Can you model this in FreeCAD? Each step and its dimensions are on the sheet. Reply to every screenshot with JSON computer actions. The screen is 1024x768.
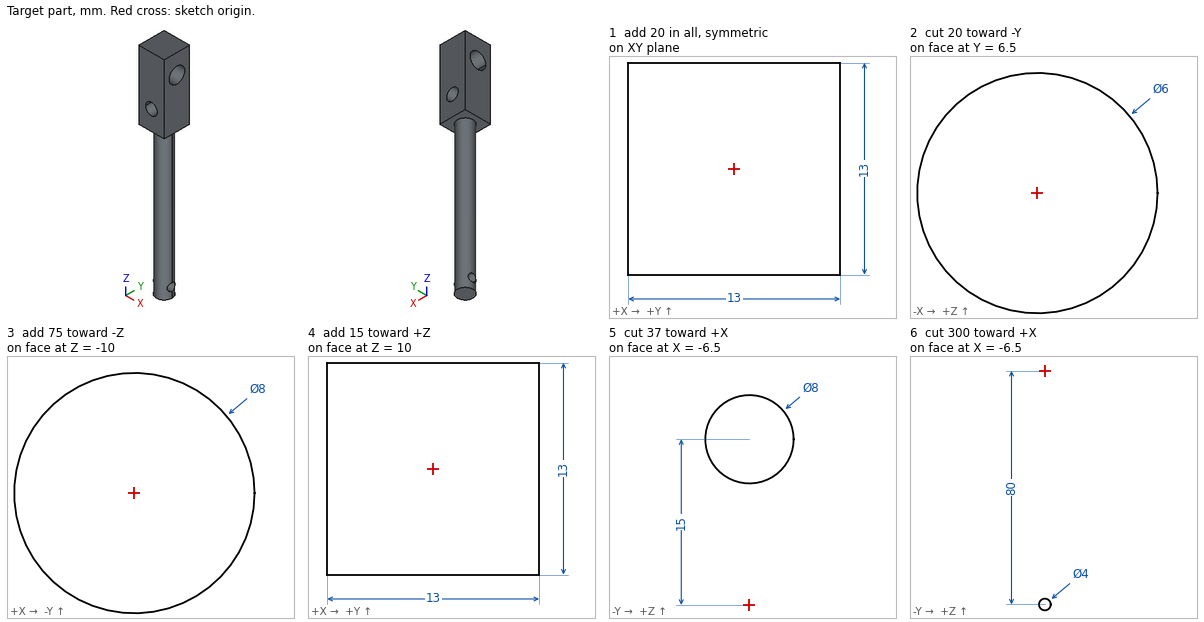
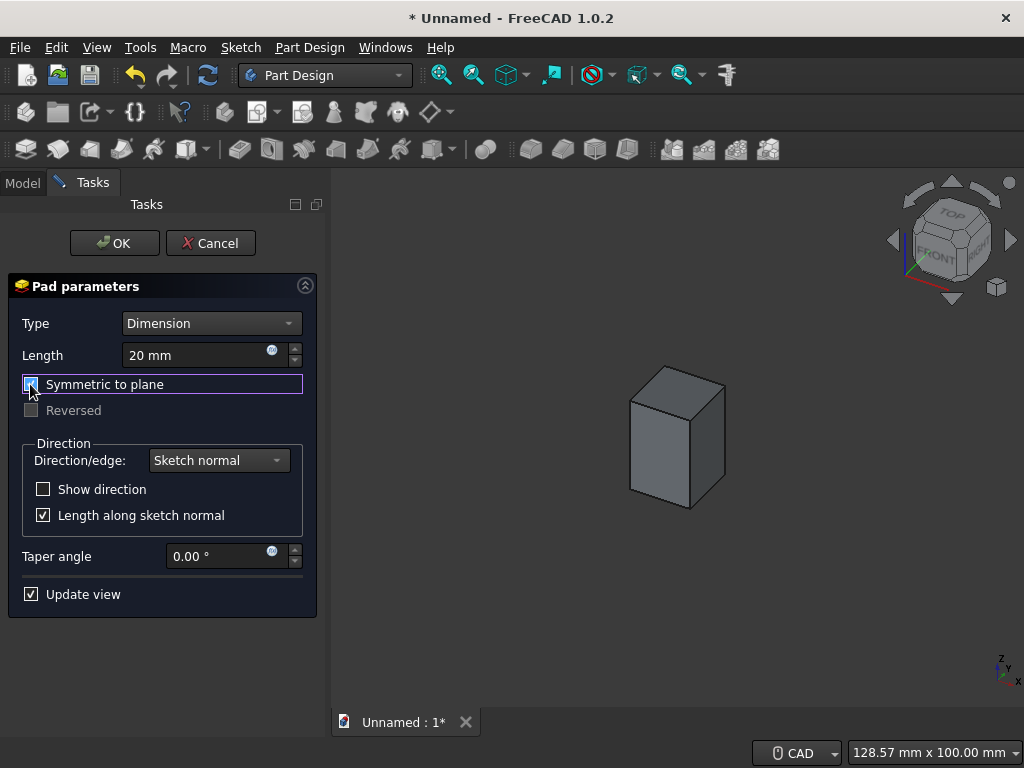
{"action": "left_click", "coordinate": [115, 243]}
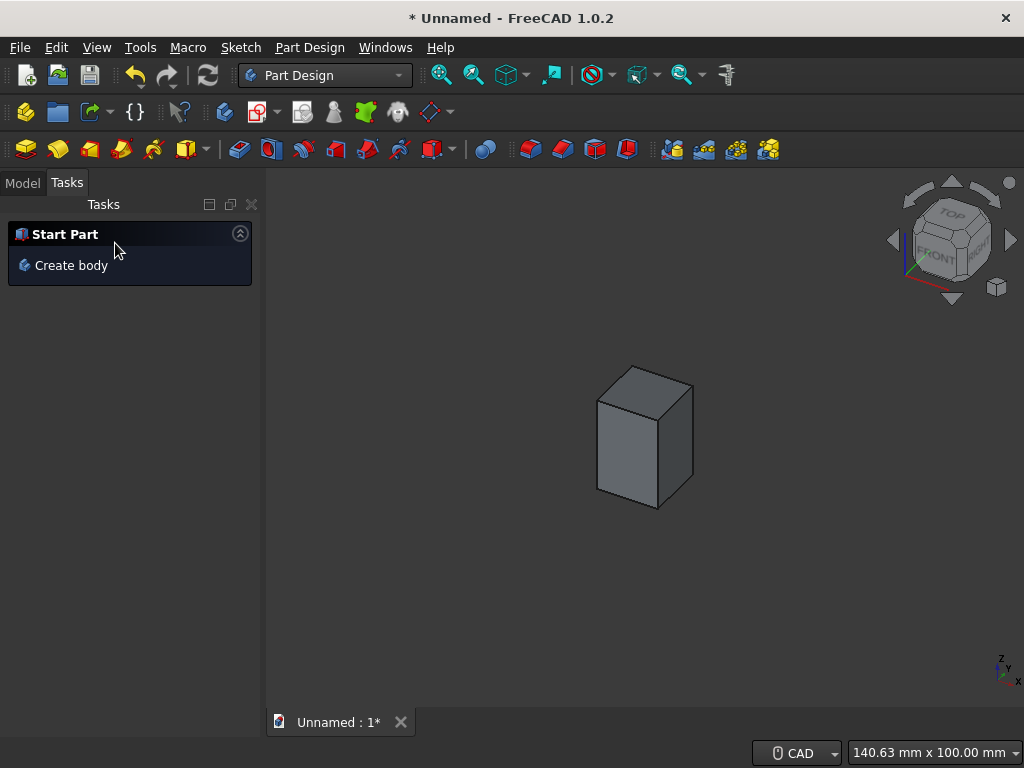
{"action": "left_click", "coordinate": [442, 76]}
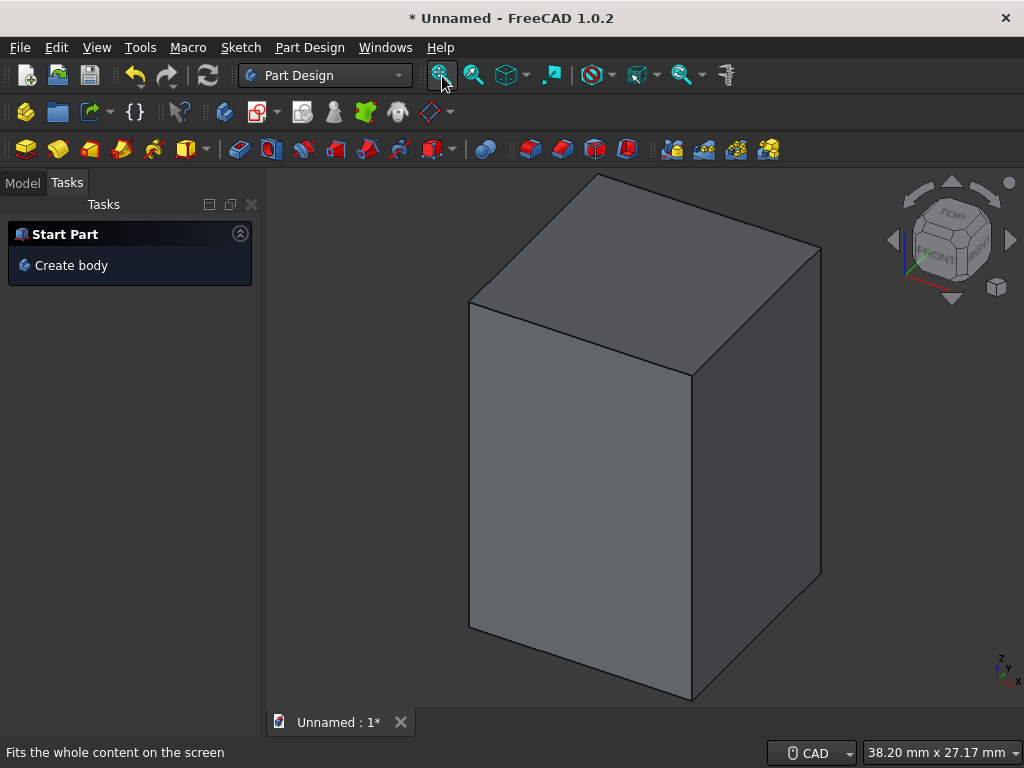
{"action": "key", "text": "4"}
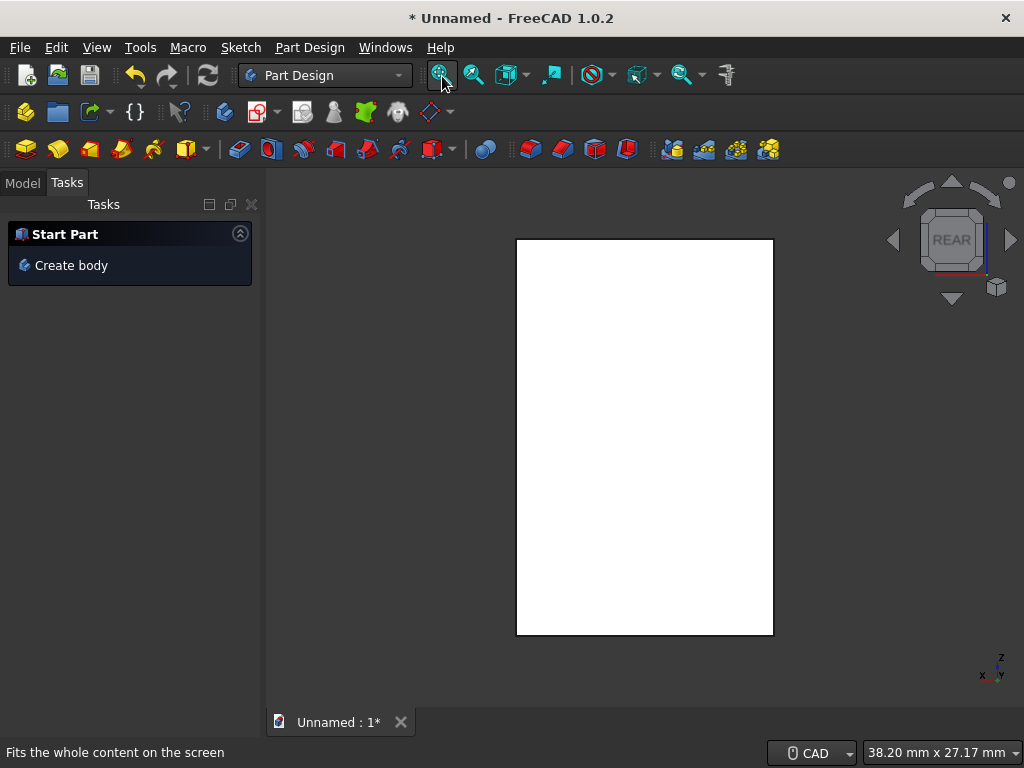
{"action": "left_click", "coordinate": [645, 380]}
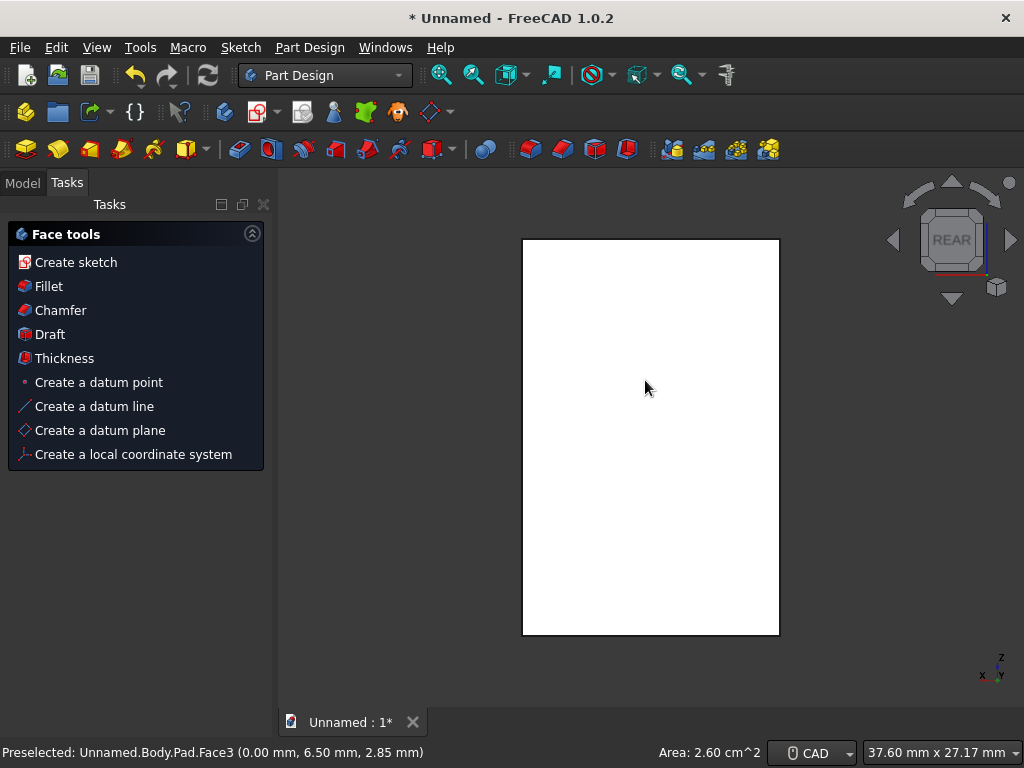
{"action": "left_click", "coordinate": [258, 112]}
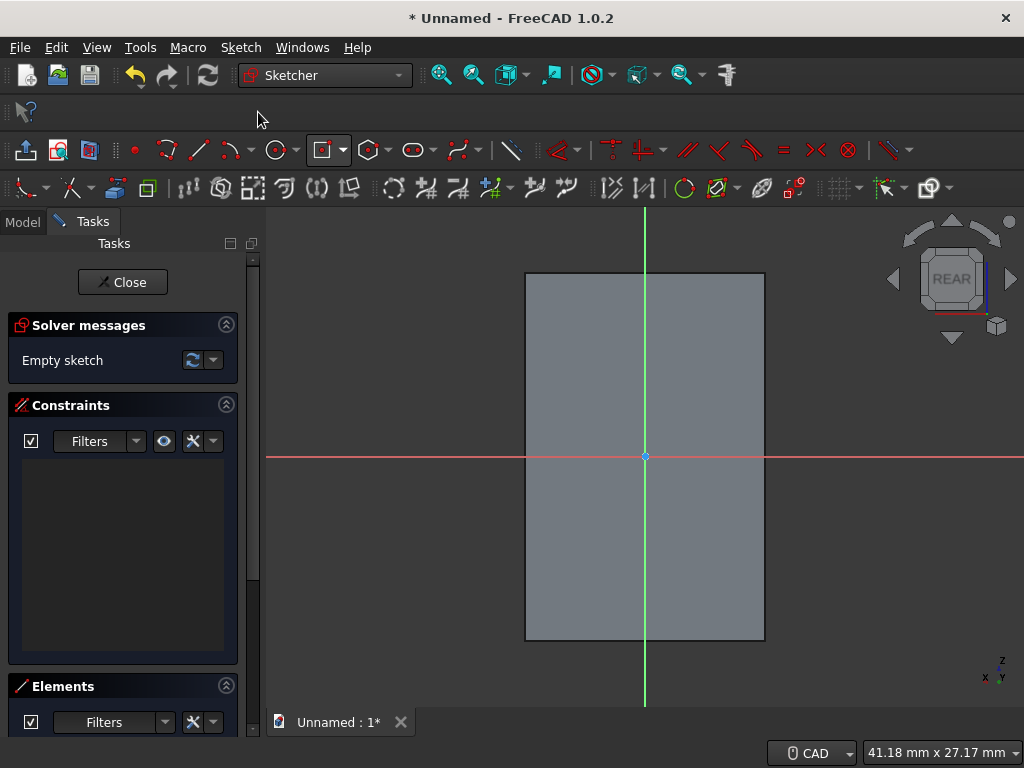
{"action": "scroll", "coordinate": [685, 457], "scroll_direction": "up", "scroll_amount": 5}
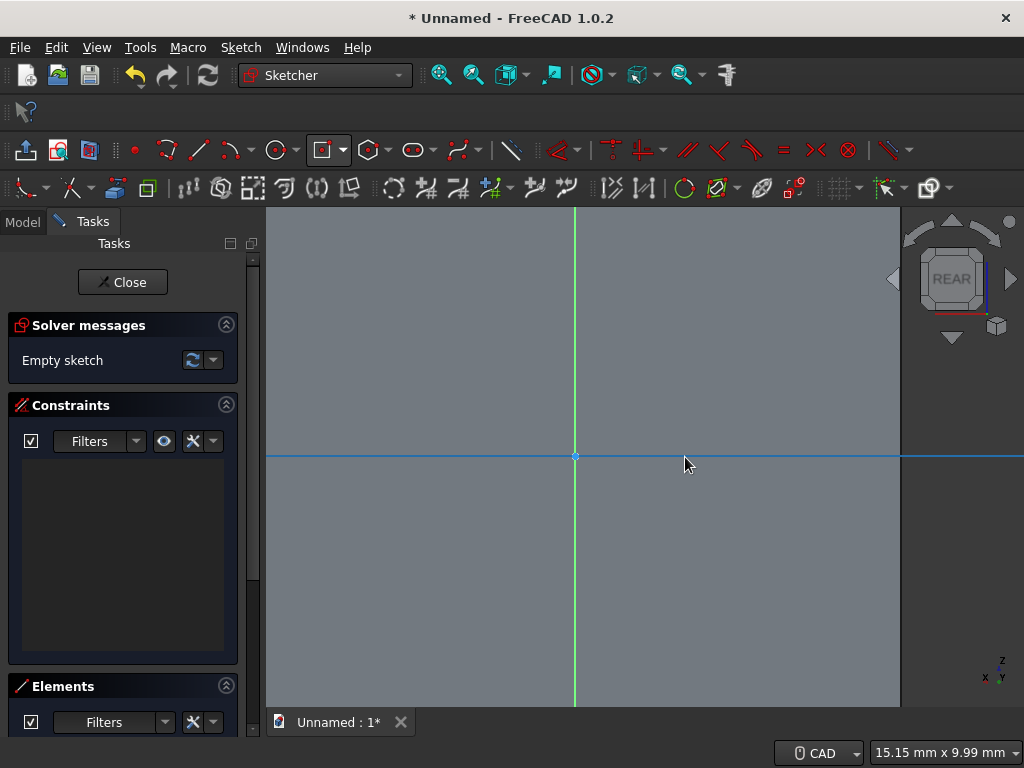
{"action": "left_click", "coordinate": [276, 150]}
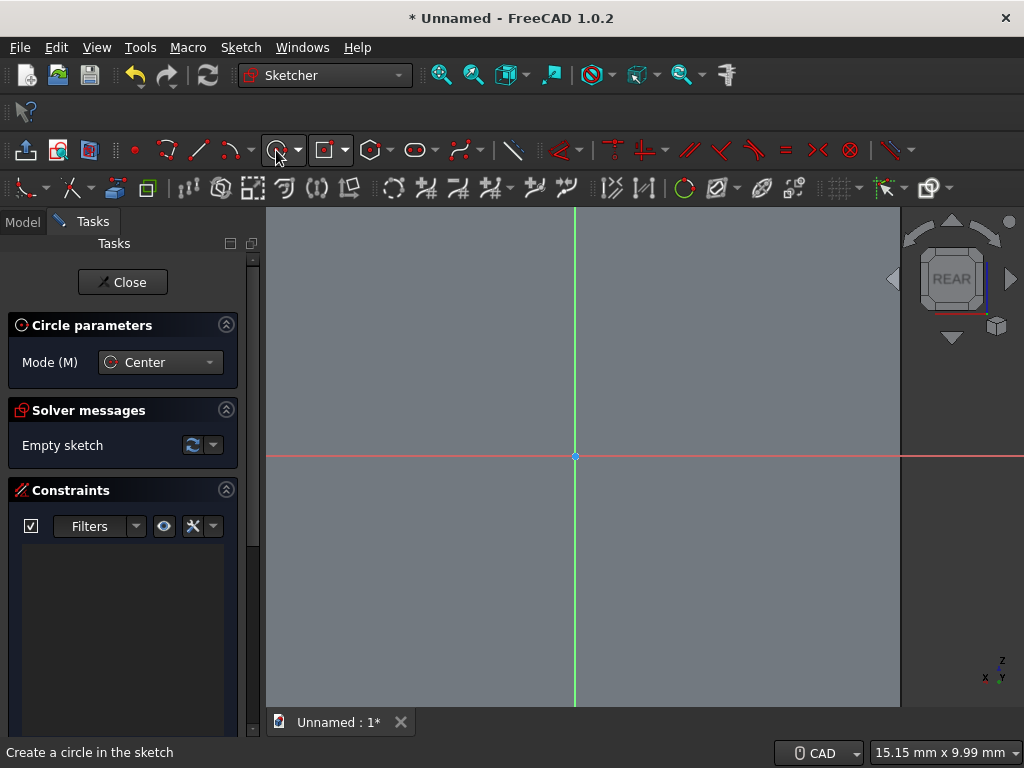
{"action": "left_click", "coordinate": [575, 456]}
{"action": "mouse_move", "coordinate": [681, 350]}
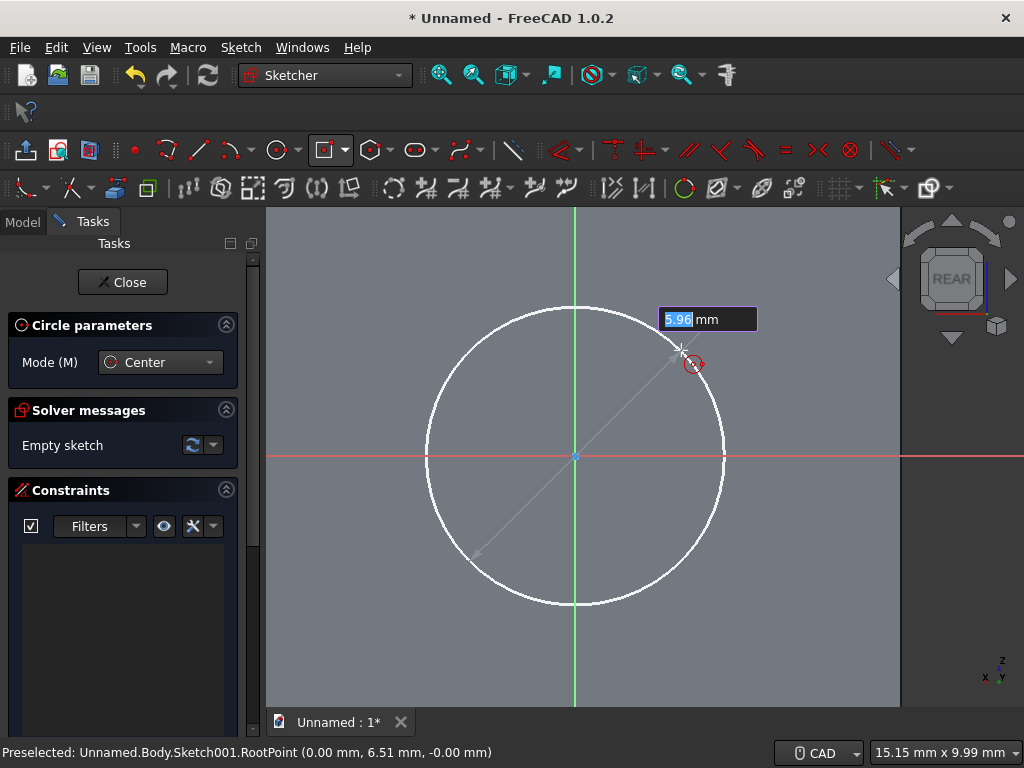
{"action": "type", "text": "6"}
{"action": "key", "text": "Return"}
{"action": "key", "text": "Escape"}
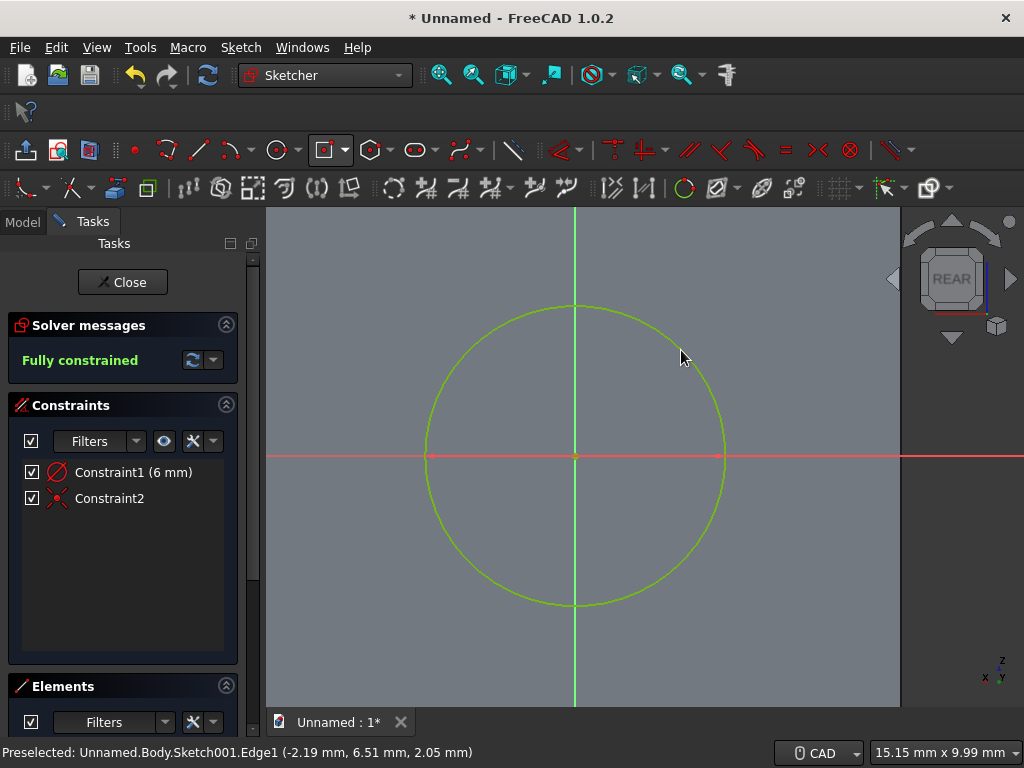
{"action": "left_click", "coordinate": [123, 282]}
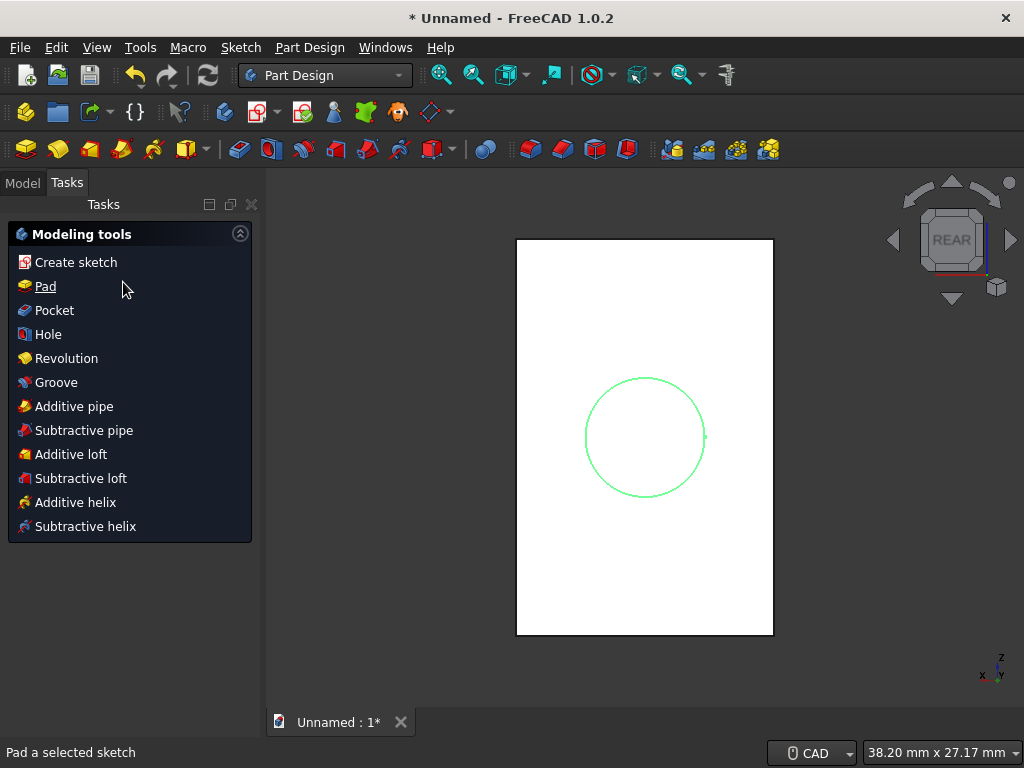
{"action": "left_click", "coordinate": [240, 150]}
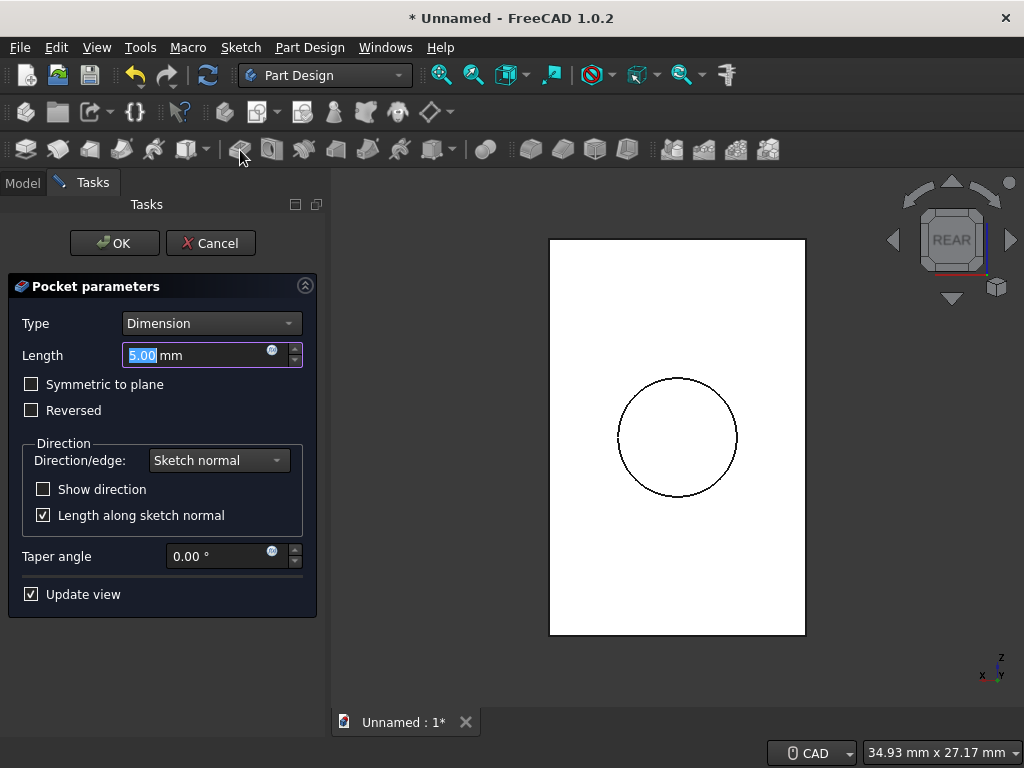
{"action": "type", "text": "20"}
{"action": "key", "text": "Tab"}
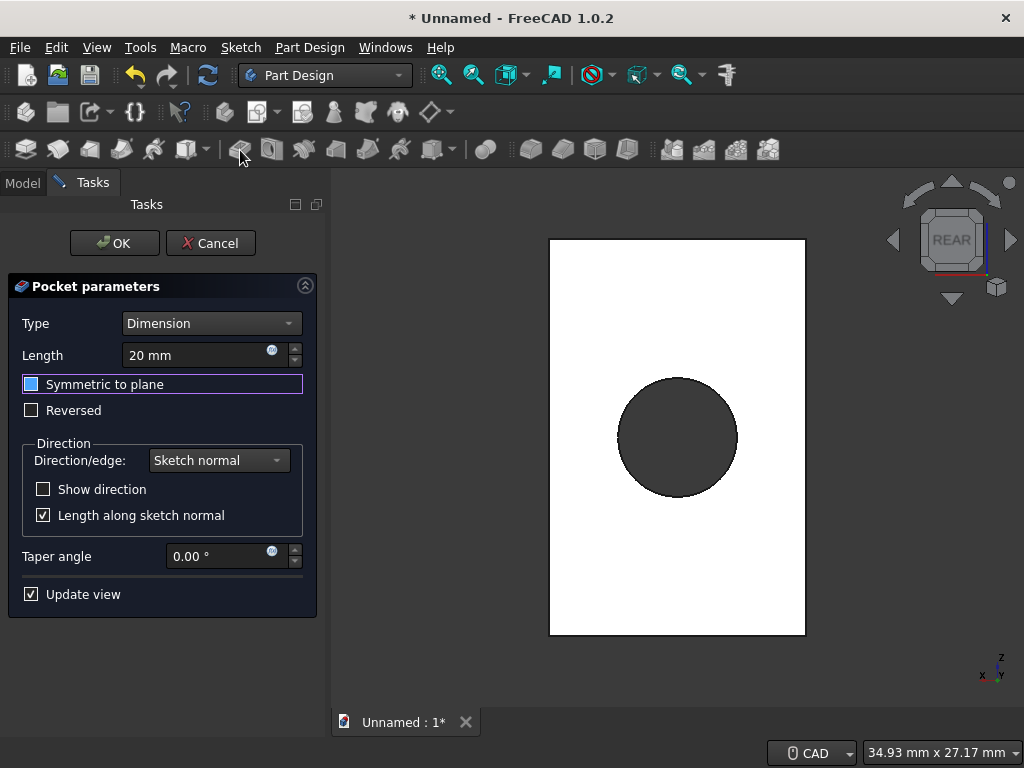
{"action": "left_click", "coordinate": [115, 243]}